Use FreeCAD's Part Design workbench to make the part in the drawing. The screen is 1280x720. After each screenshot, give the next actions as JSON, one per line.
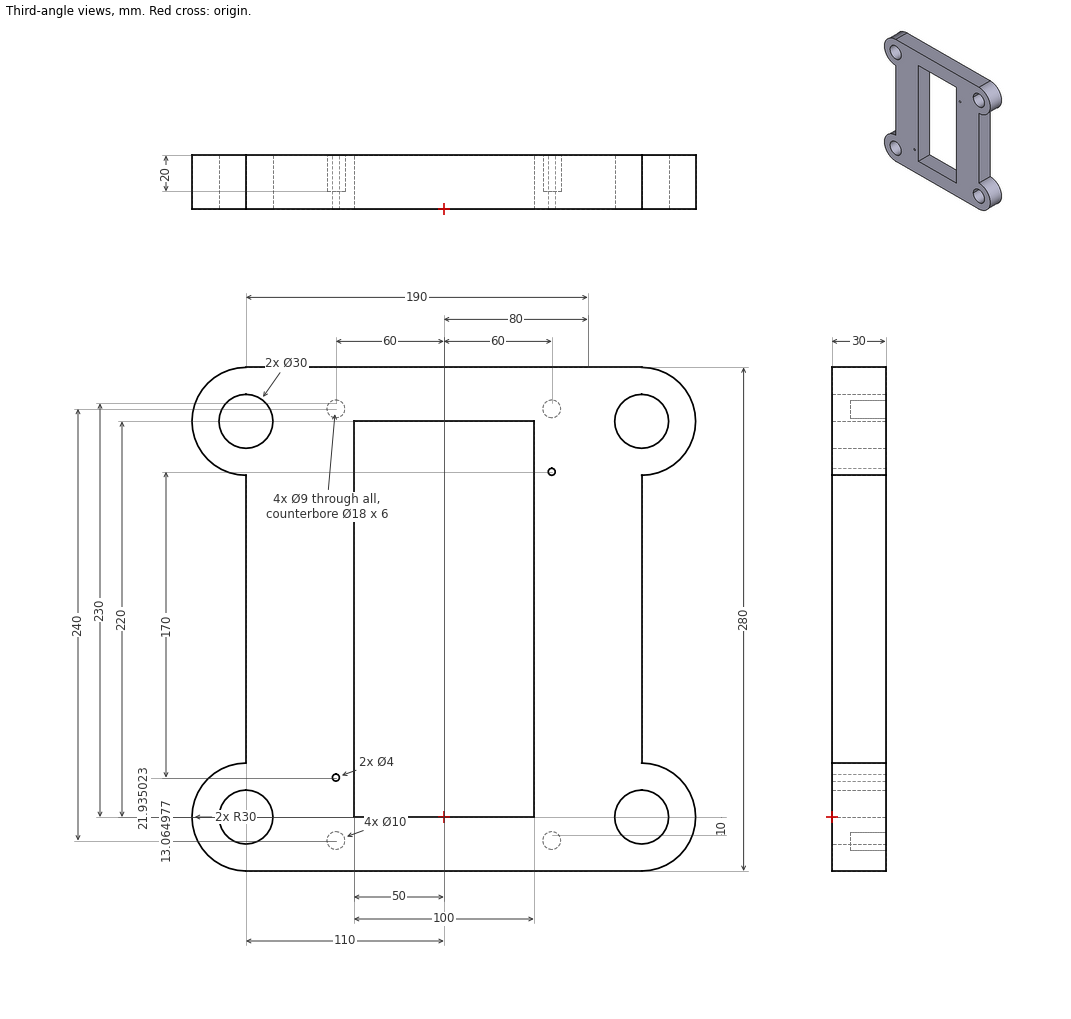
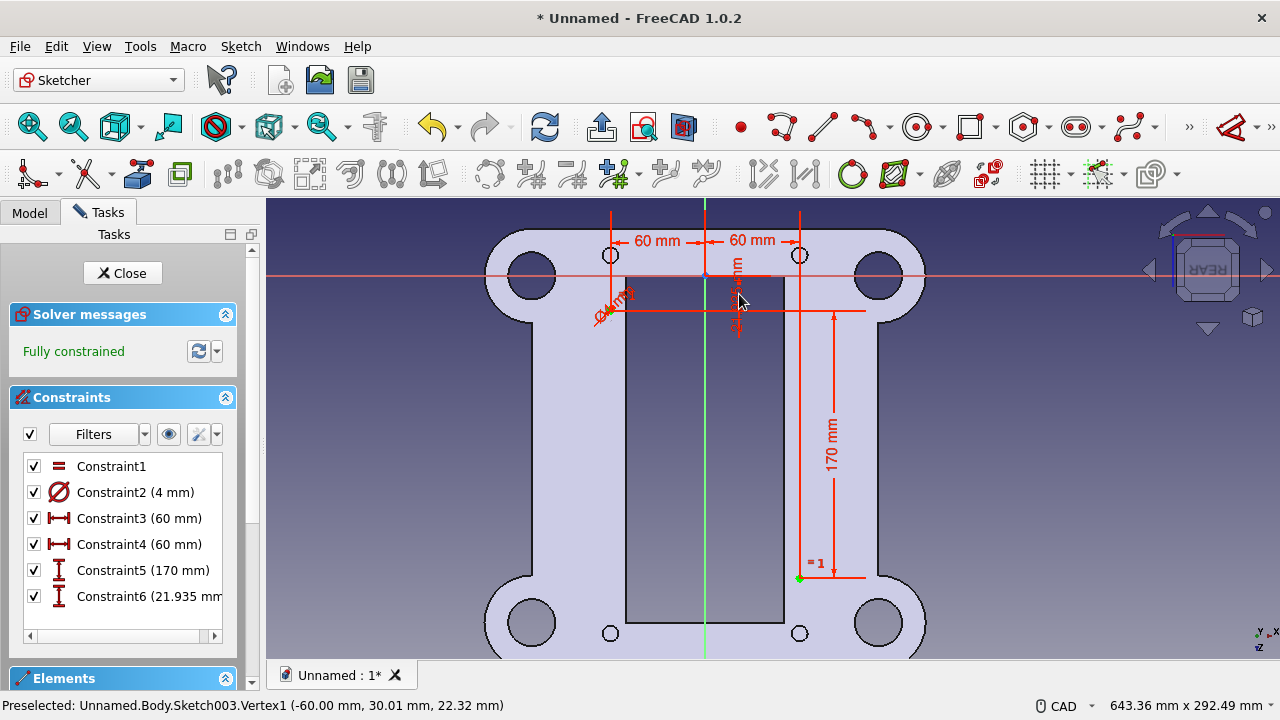
{"action": "left_click", "coordinate": [123, 273]}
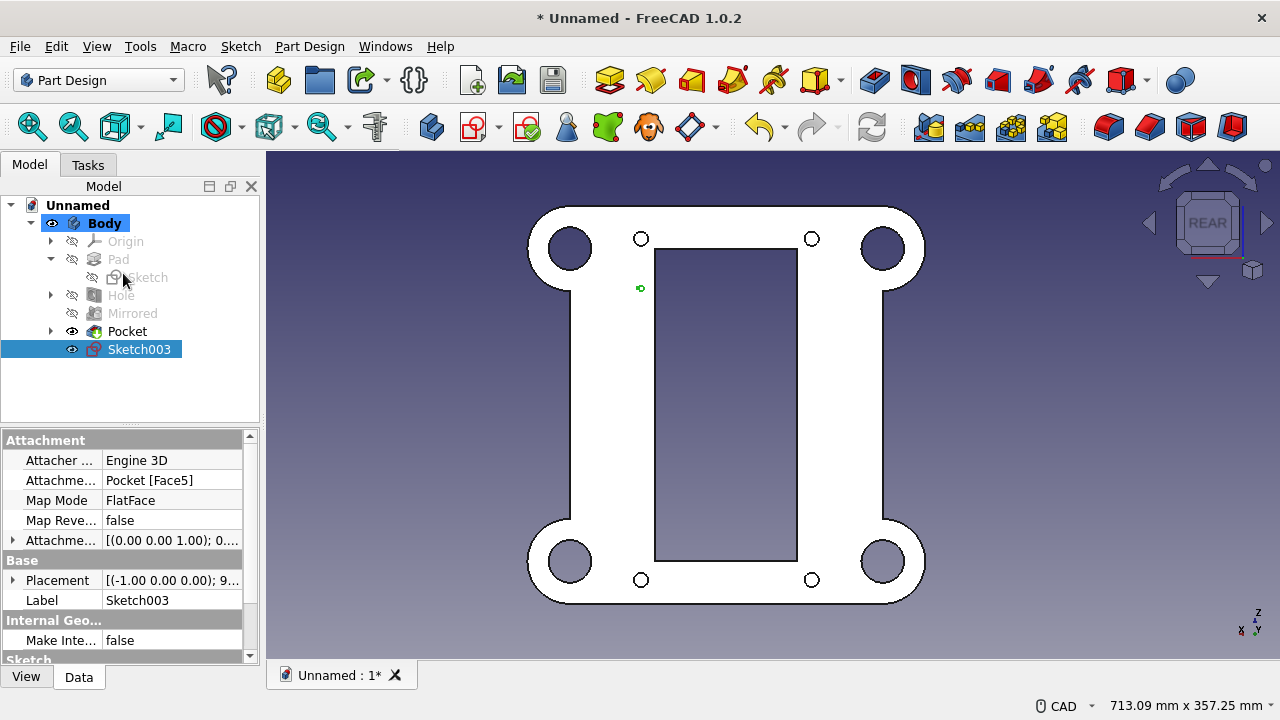
{"action": "left_click", "coordinate": [875, 80]}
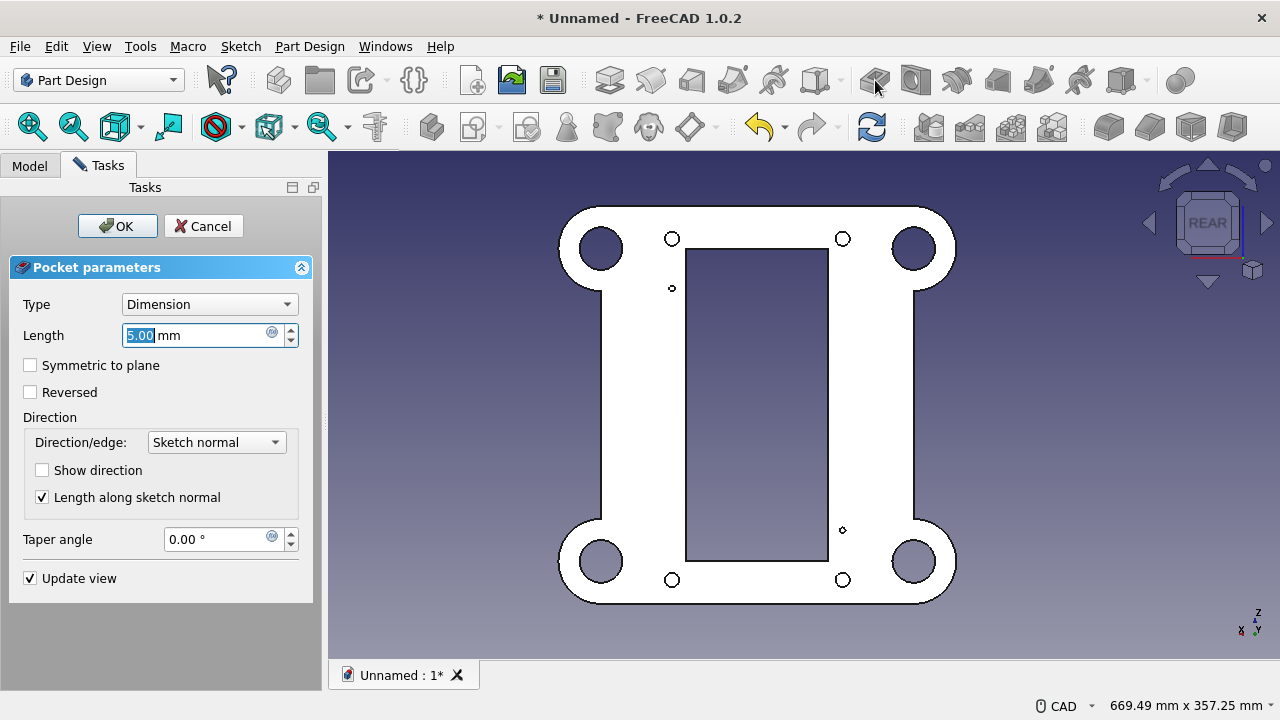
{"action": "left_click", "coordinate": [210, 304]}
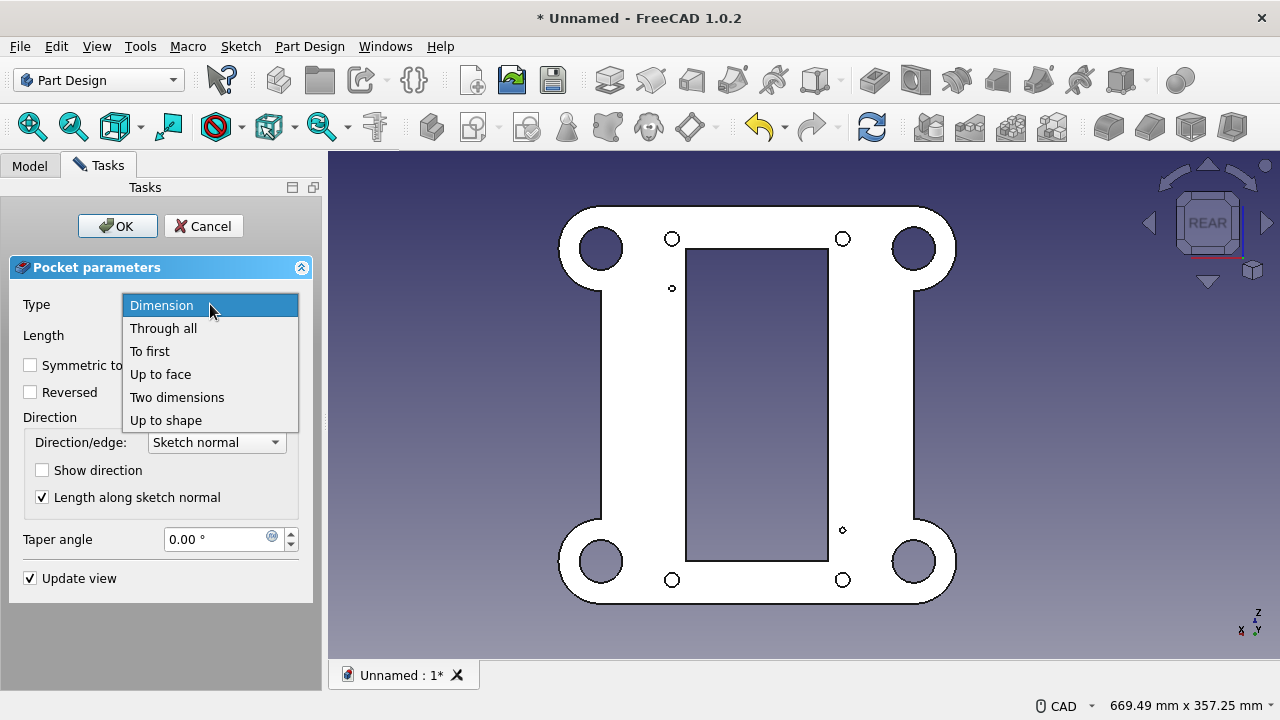
{"action": "left_click", "coordinate": [208, 328]}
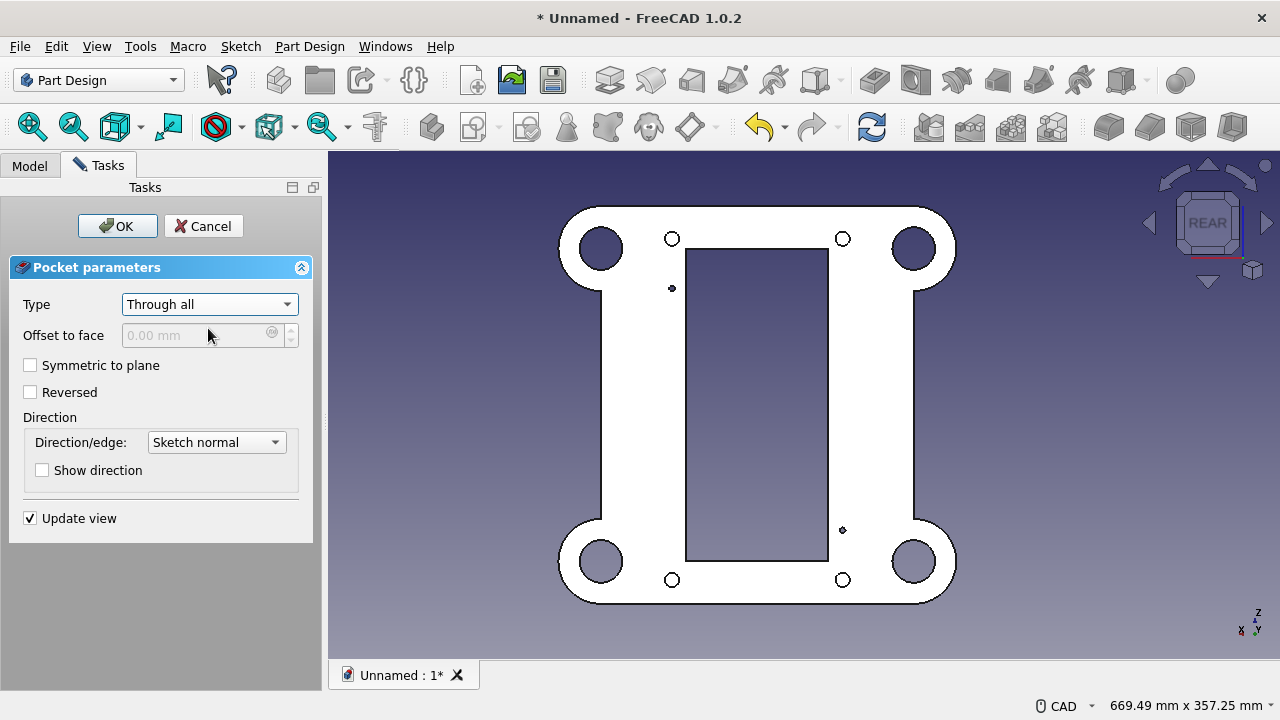
{"action": "left_click", "coordinate": [118, 226]}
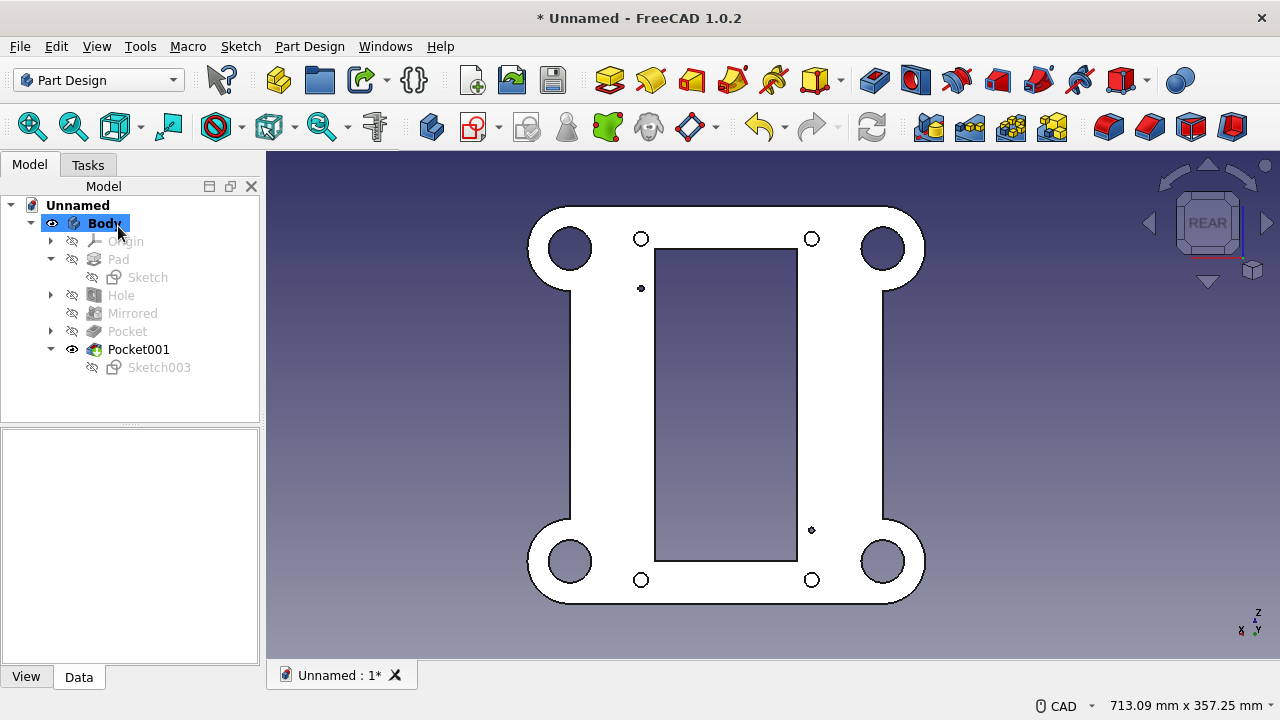
{"action": "key", "text": "0"}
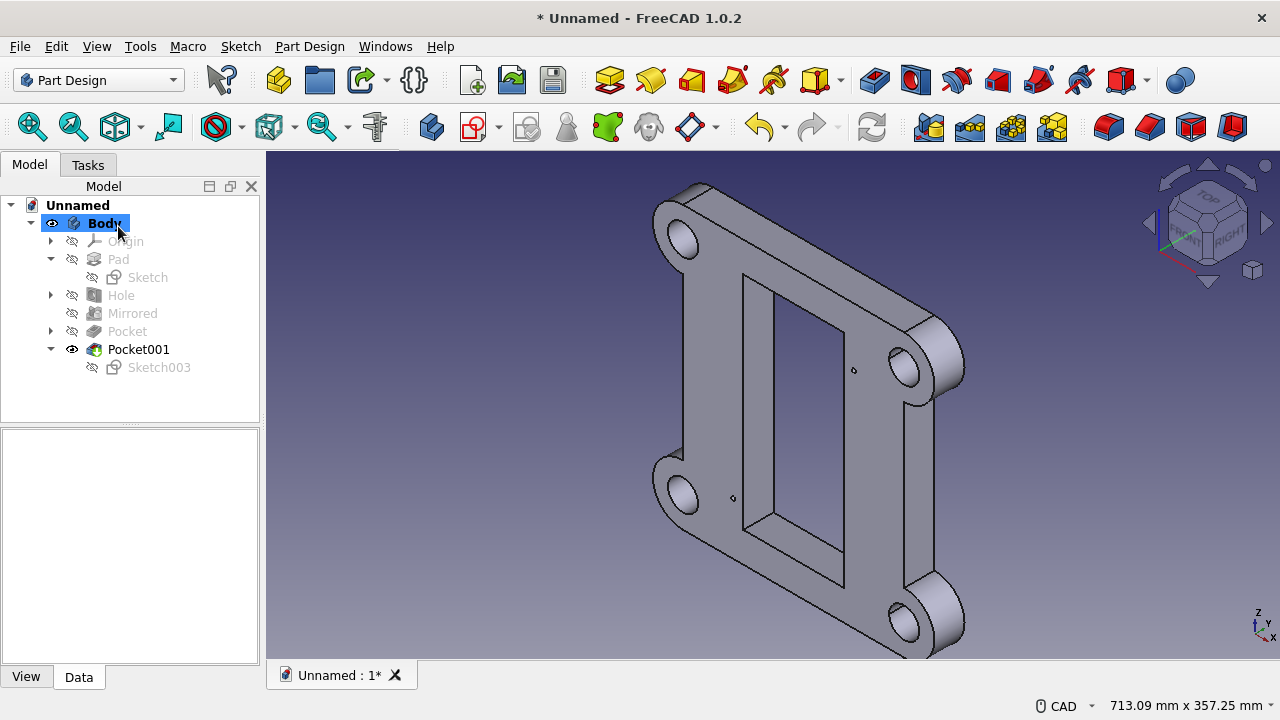
{"action": "key", "text": "v f"}